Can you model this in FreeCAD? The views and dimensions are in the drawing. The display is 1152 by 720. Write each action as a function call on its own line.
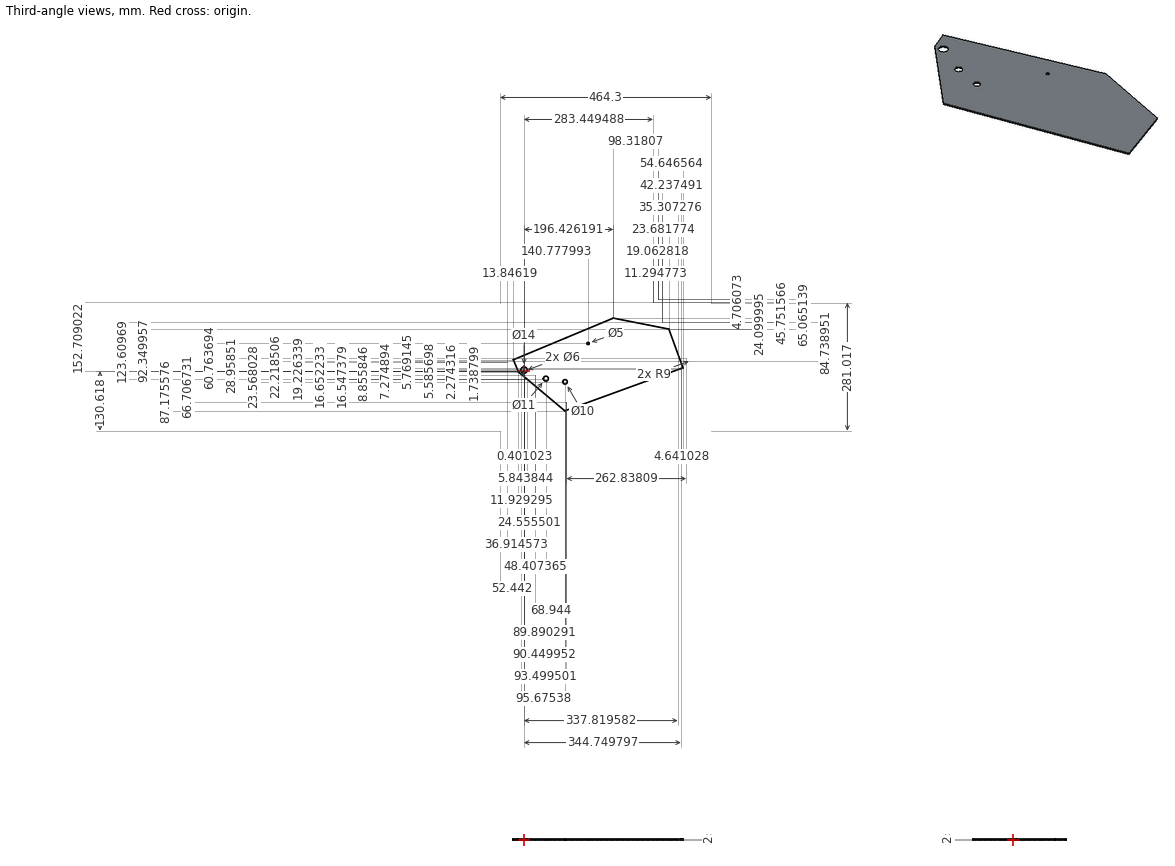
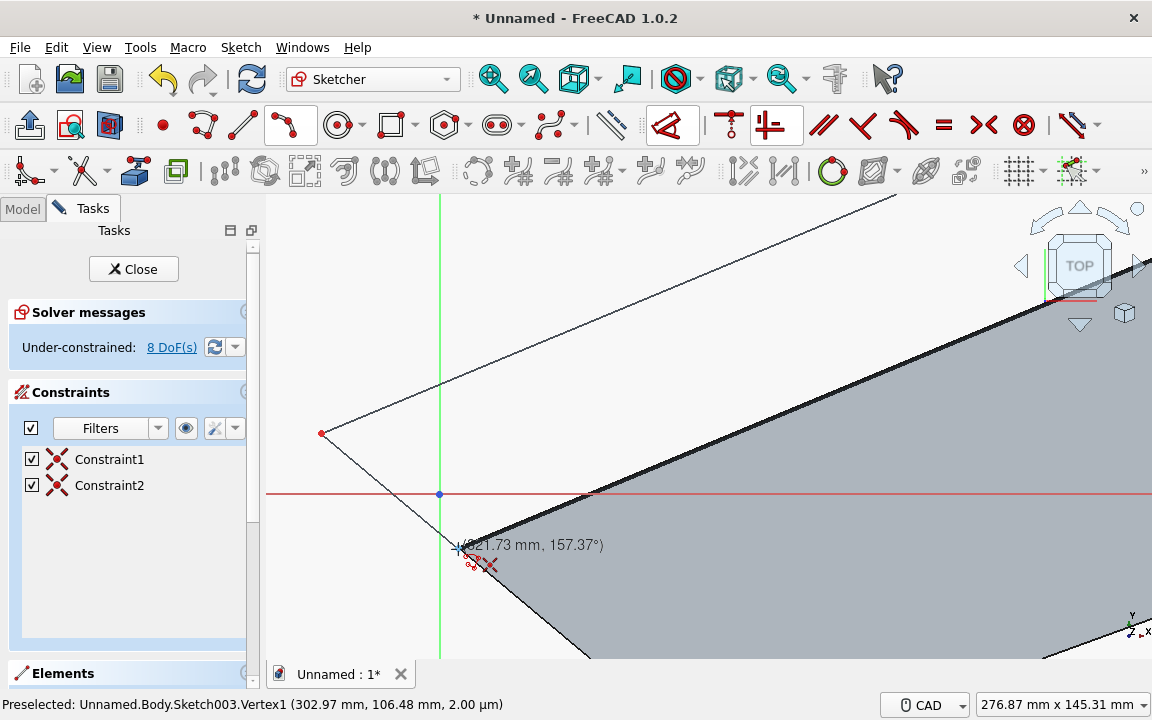
click(458, 549)
key(Escape)
key(Escape)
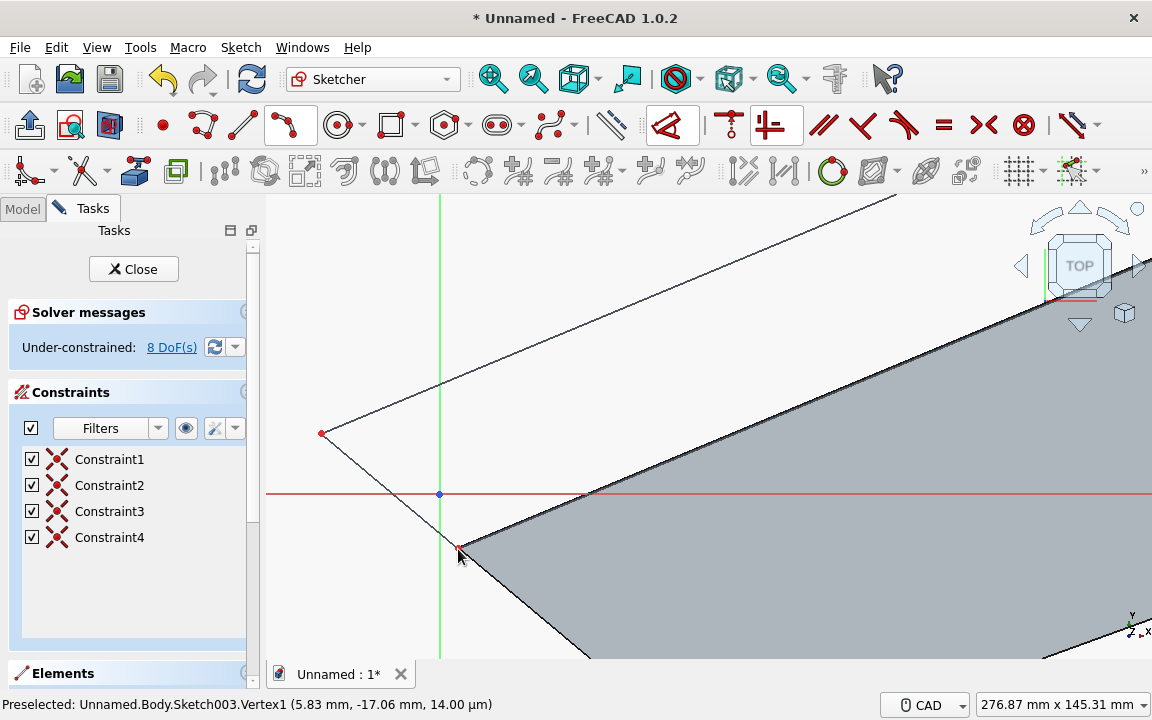
scroll(458, 549, up, 4)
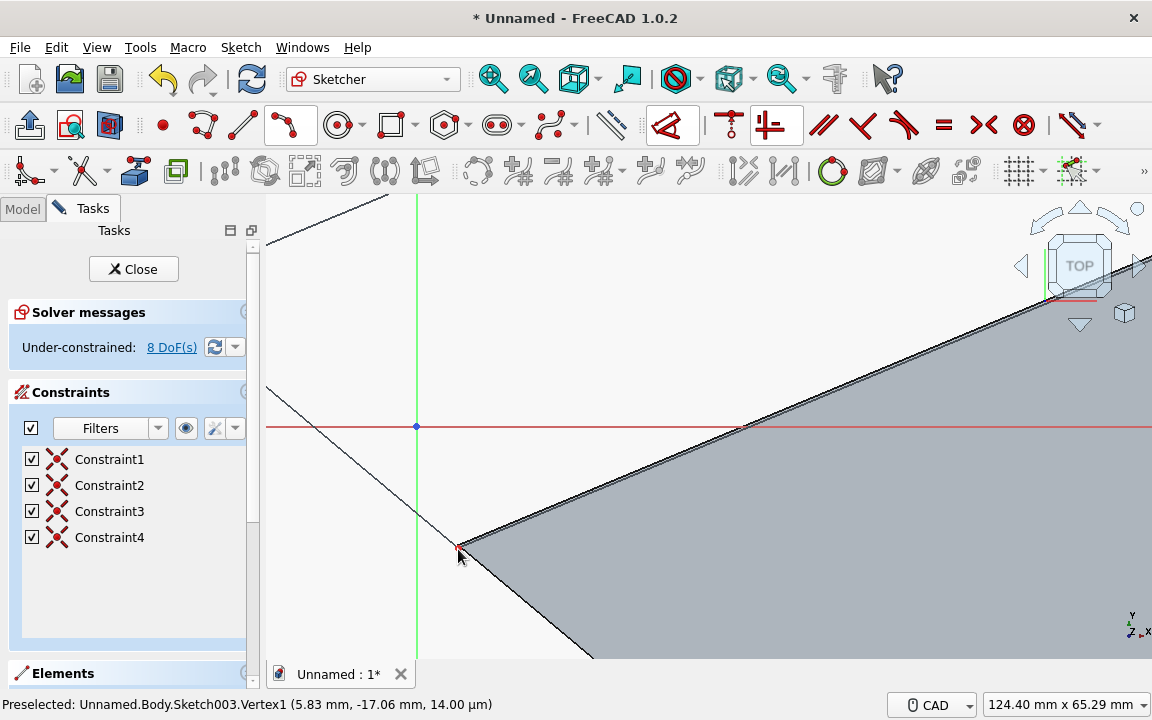
click(458, 548)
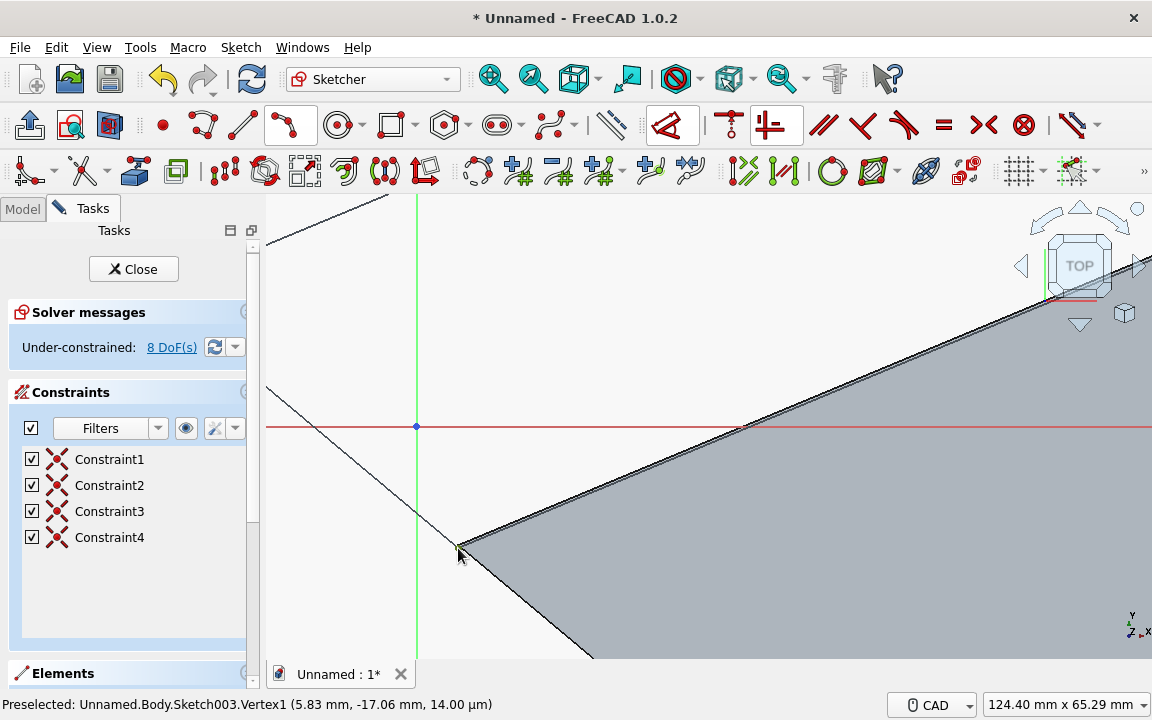
key(l)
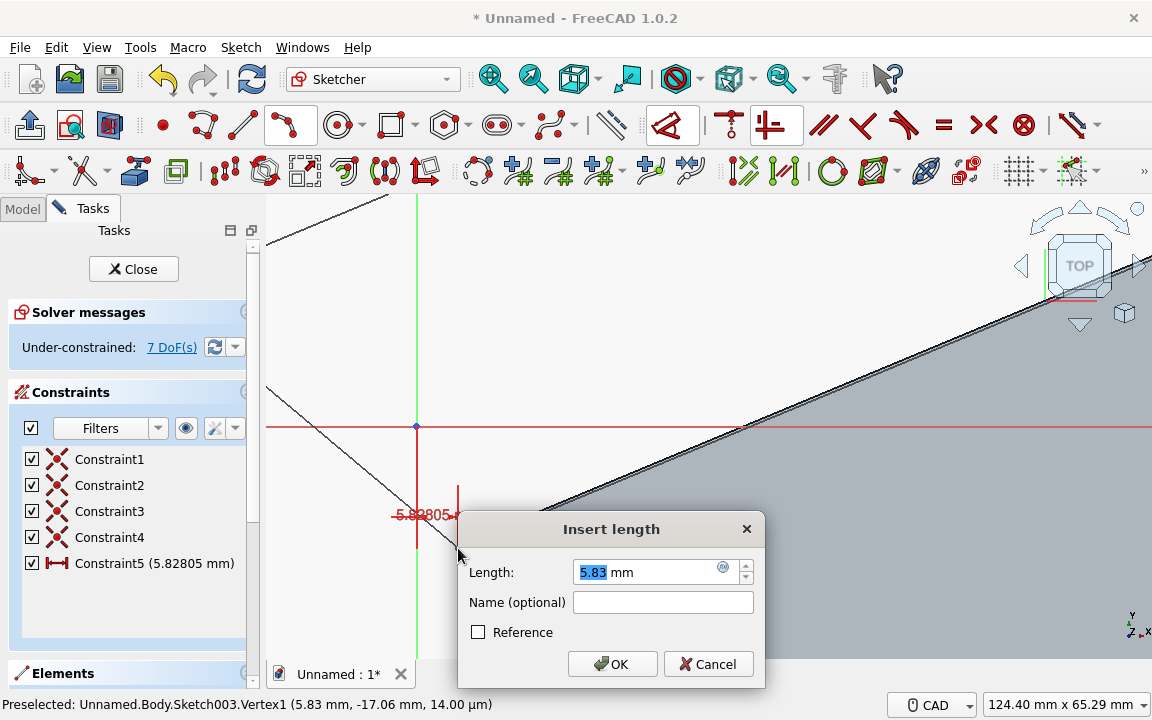
text(5.843844)
key(Return)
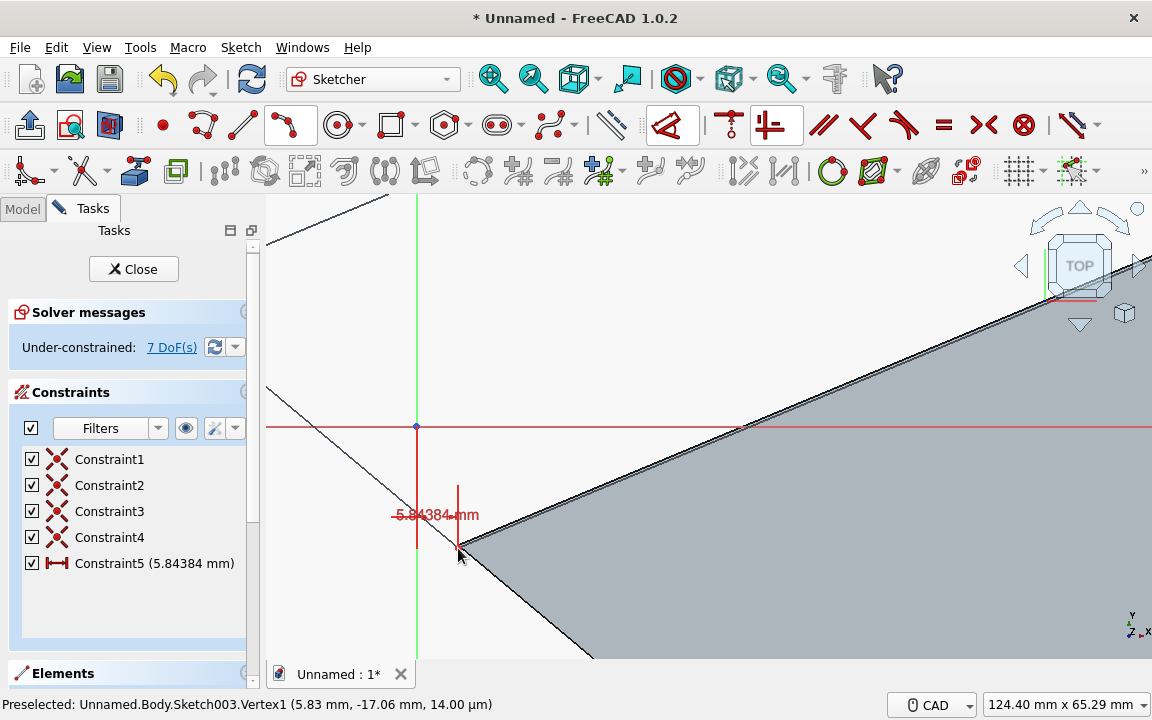
scroll(458, 549, down, 8)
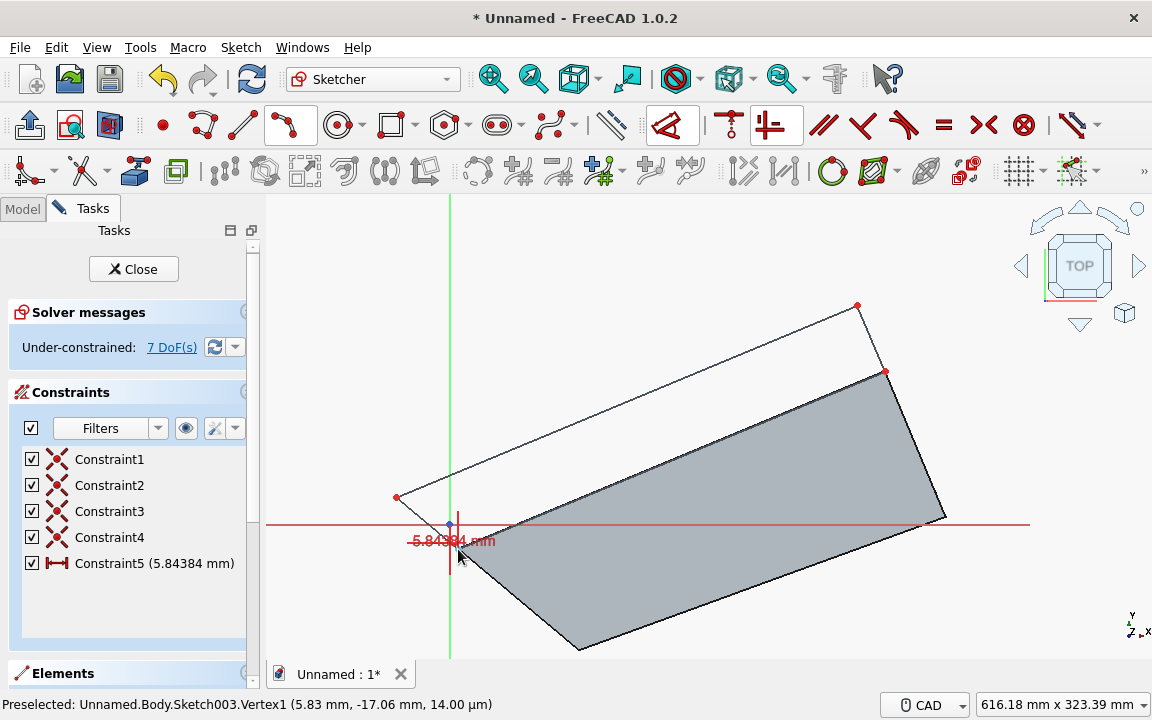
scroll(458, 549, up, 3)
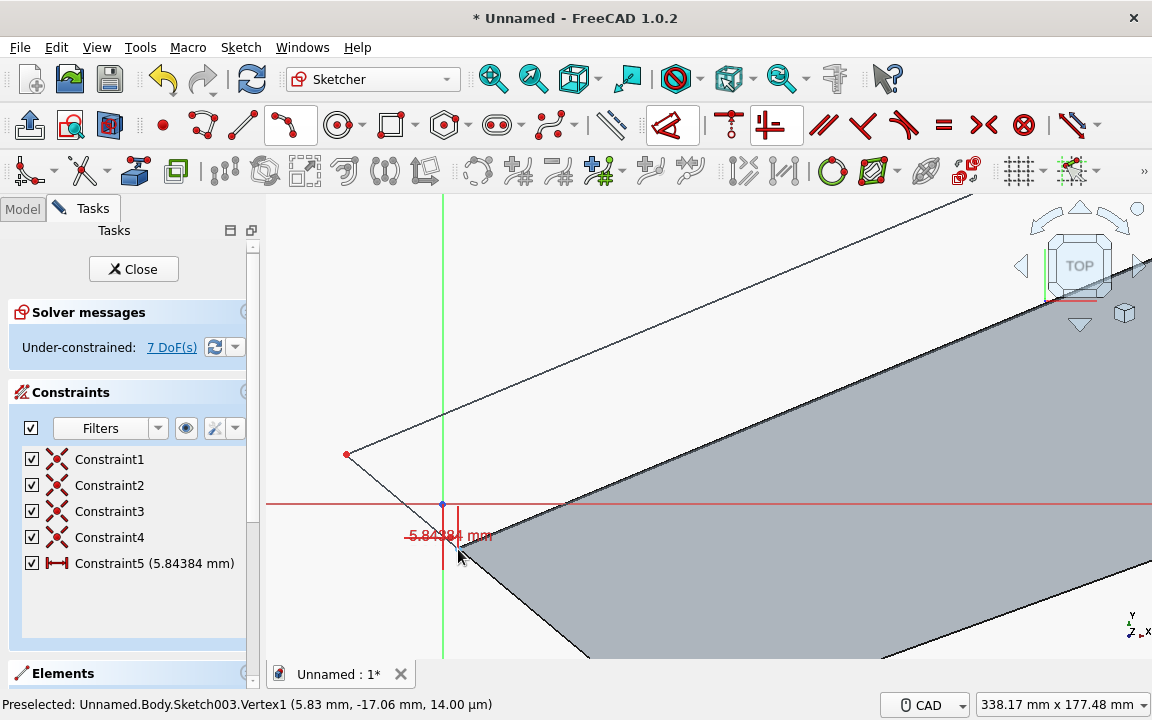
click(458, 549)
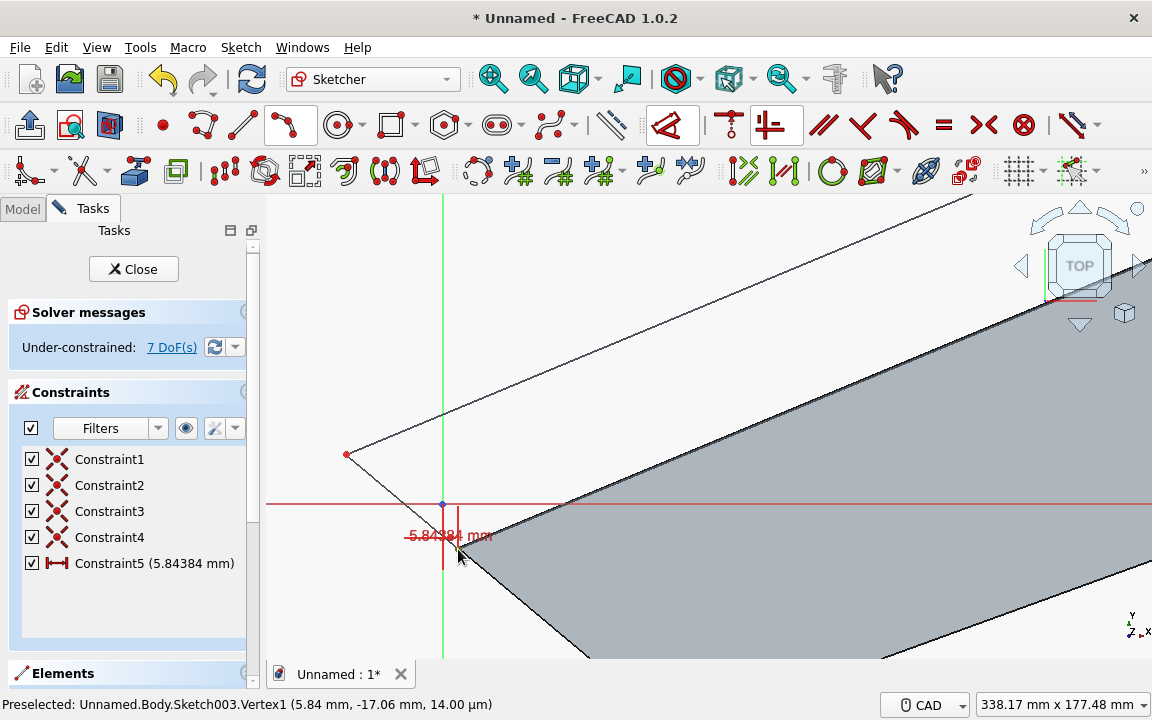
click(694, 126)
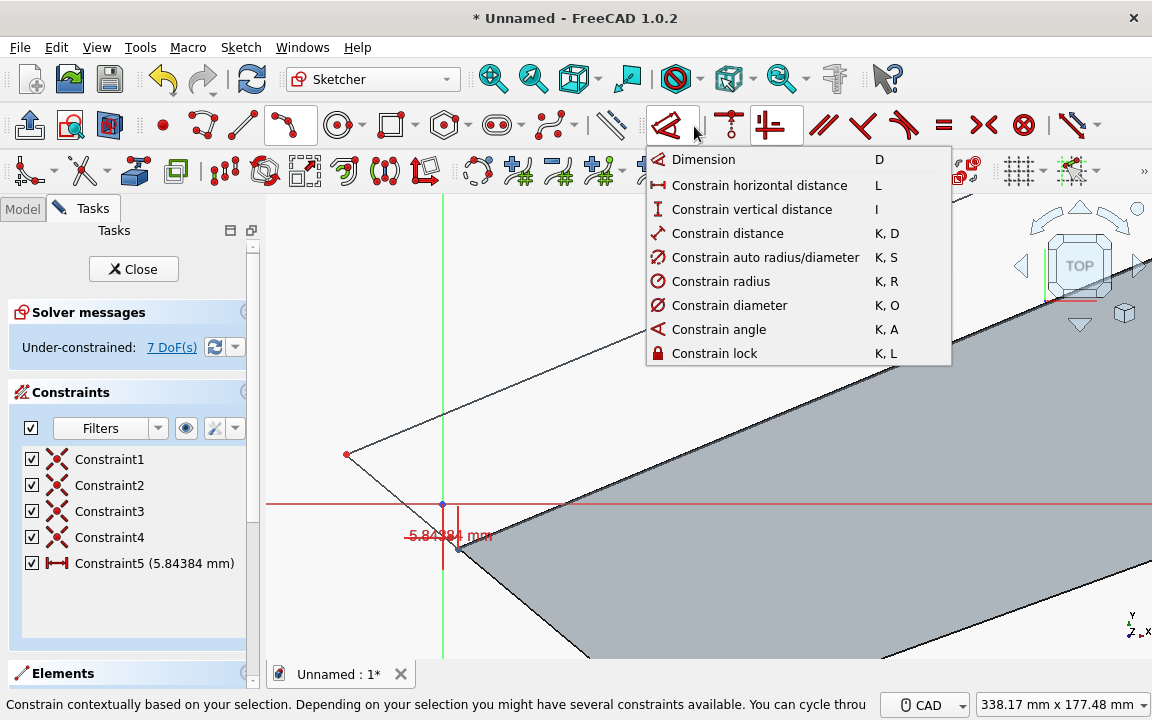
click(799, 209)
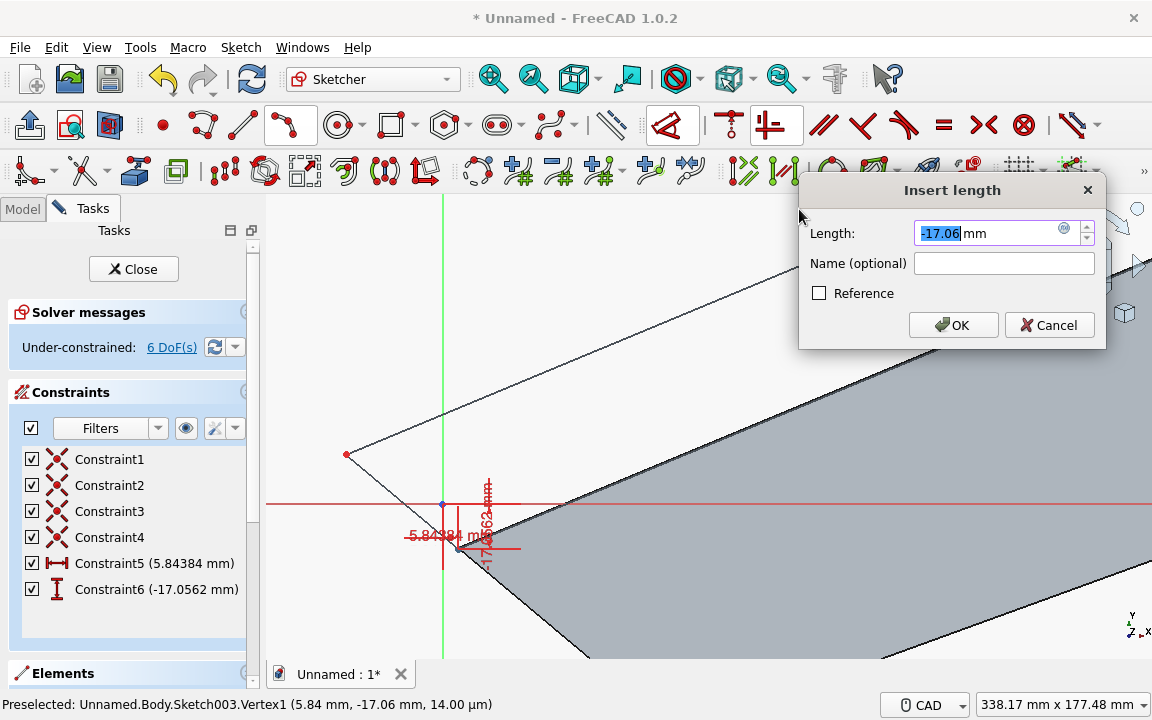
text(-16.652233)
key(Return)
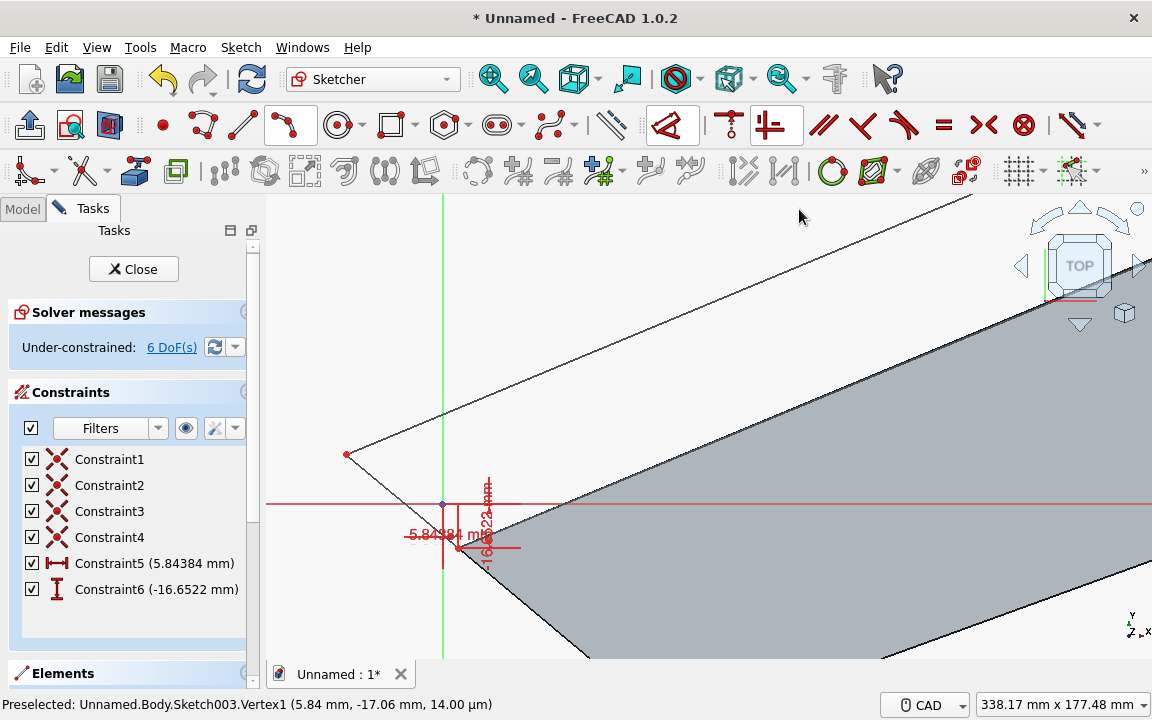
click(346, 455)